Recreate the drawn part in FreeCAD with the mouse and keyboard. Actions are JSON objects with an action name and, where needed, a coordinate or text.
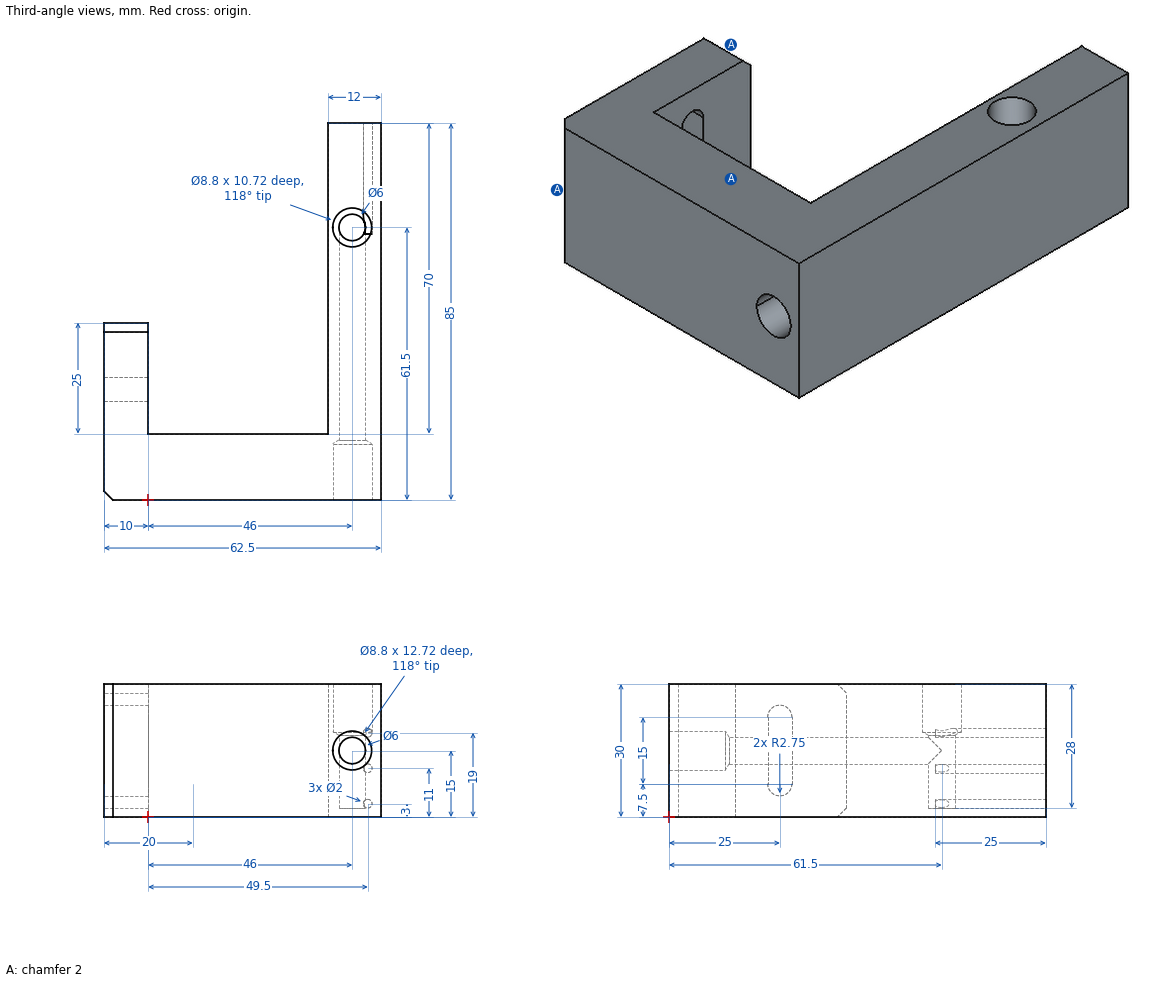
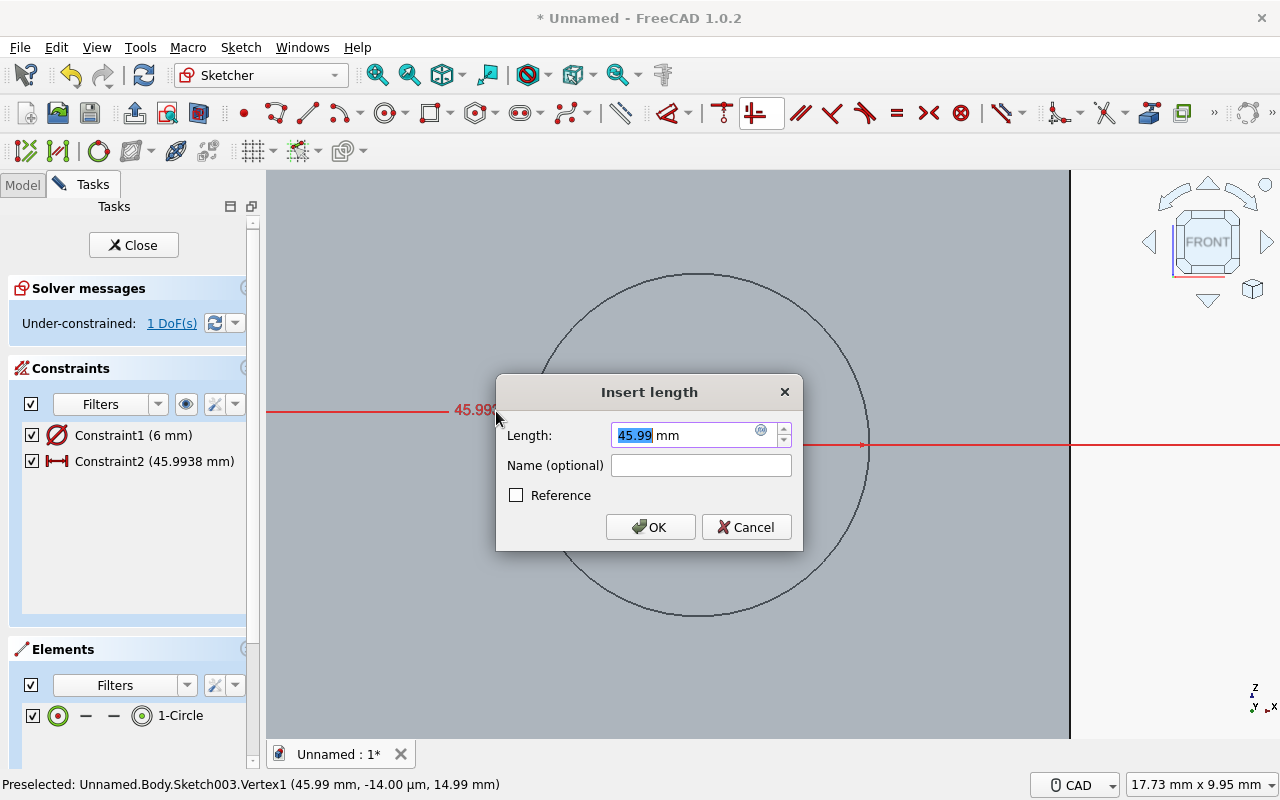
{"action": "type", "text": "46"}
{"action": "key", "text": "Return"}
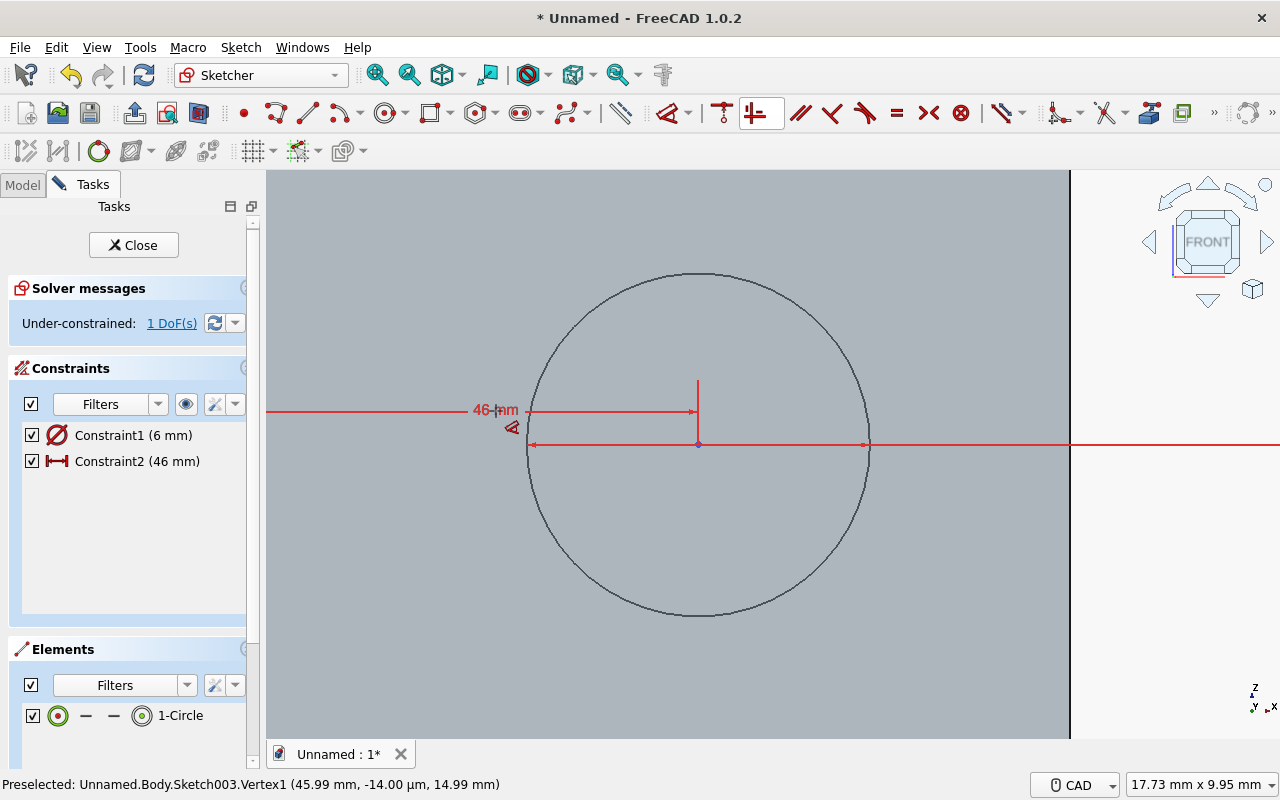
{"action": "left_click", "coordinate": [698, 445]}
{"action": "left_click", "coordinate": [732, 578]}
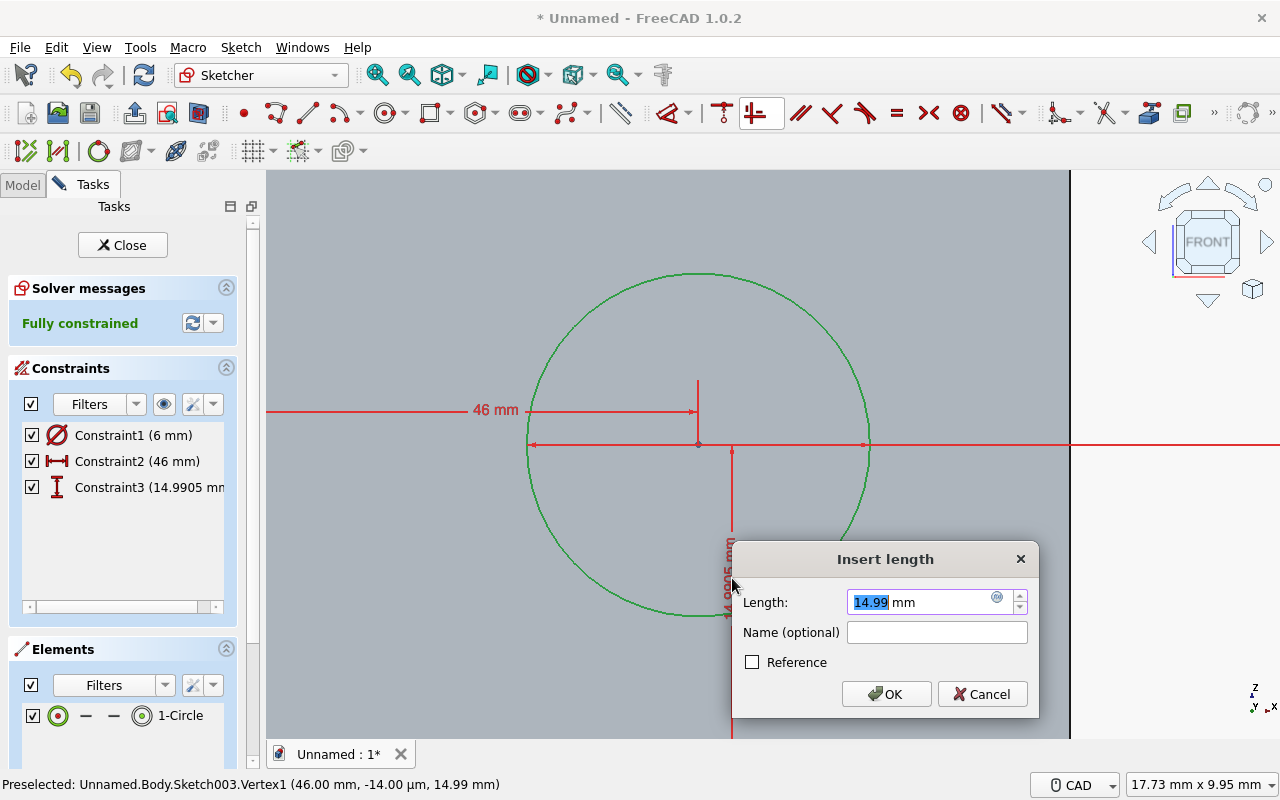
{"action": "type", "text": "15"}
{"action": "key", "text": "Return"}
{"action": "key", "text": "Escape"}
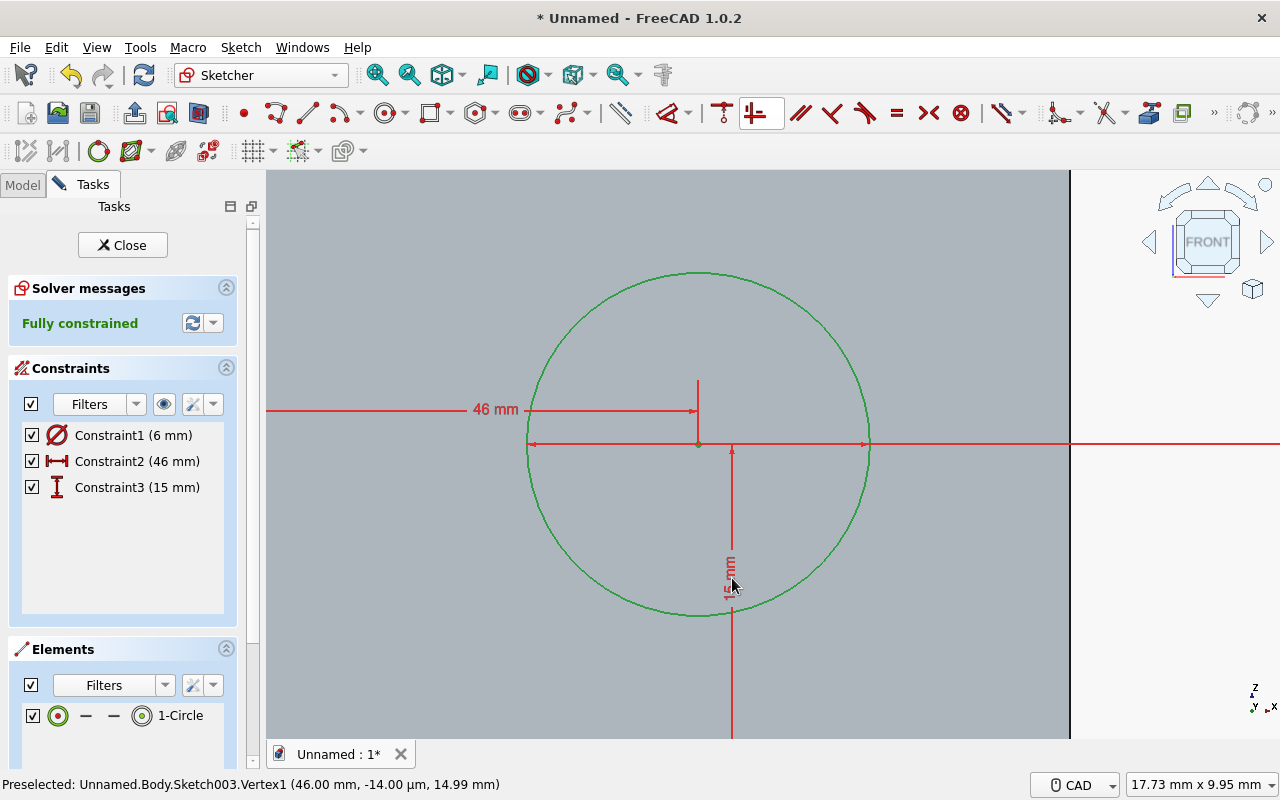
{"action": "left_click", "coordinate": [123, 245]}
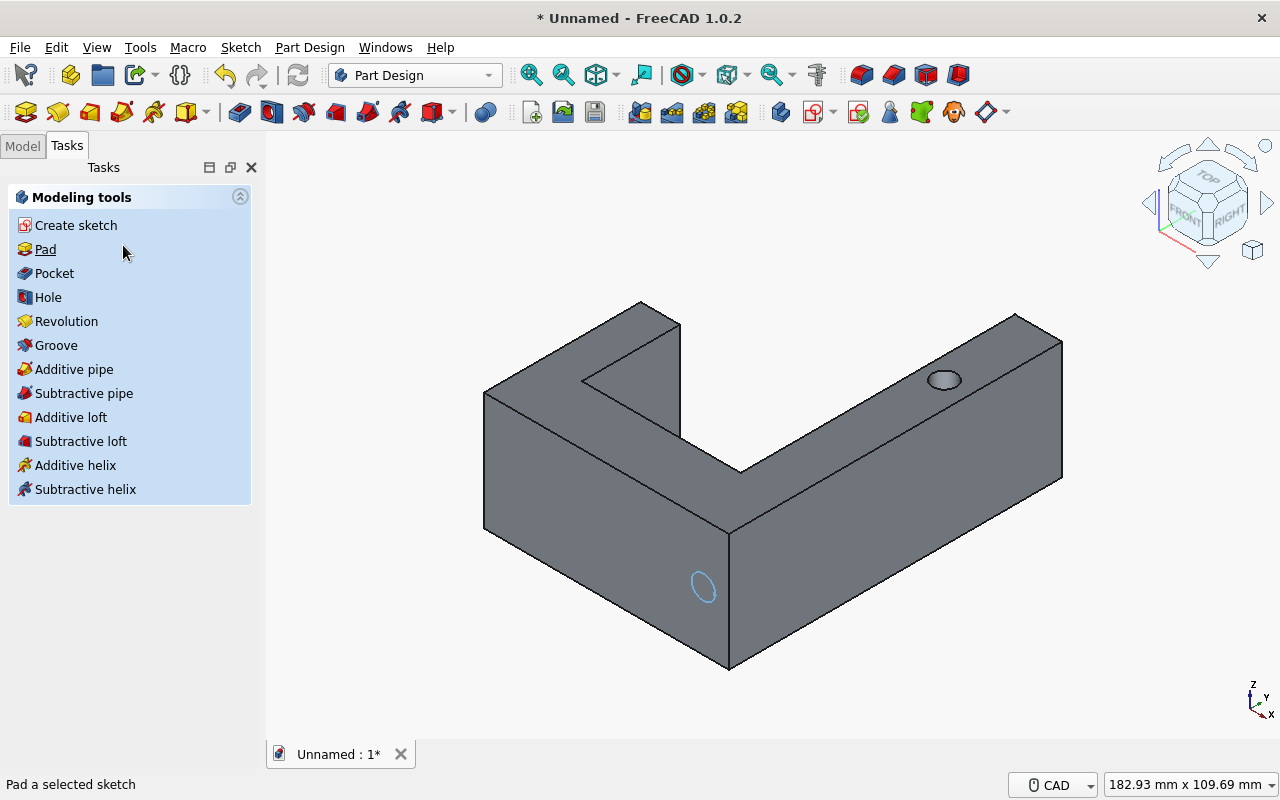
{"action": "left_click", "coordinate": [240, 112]}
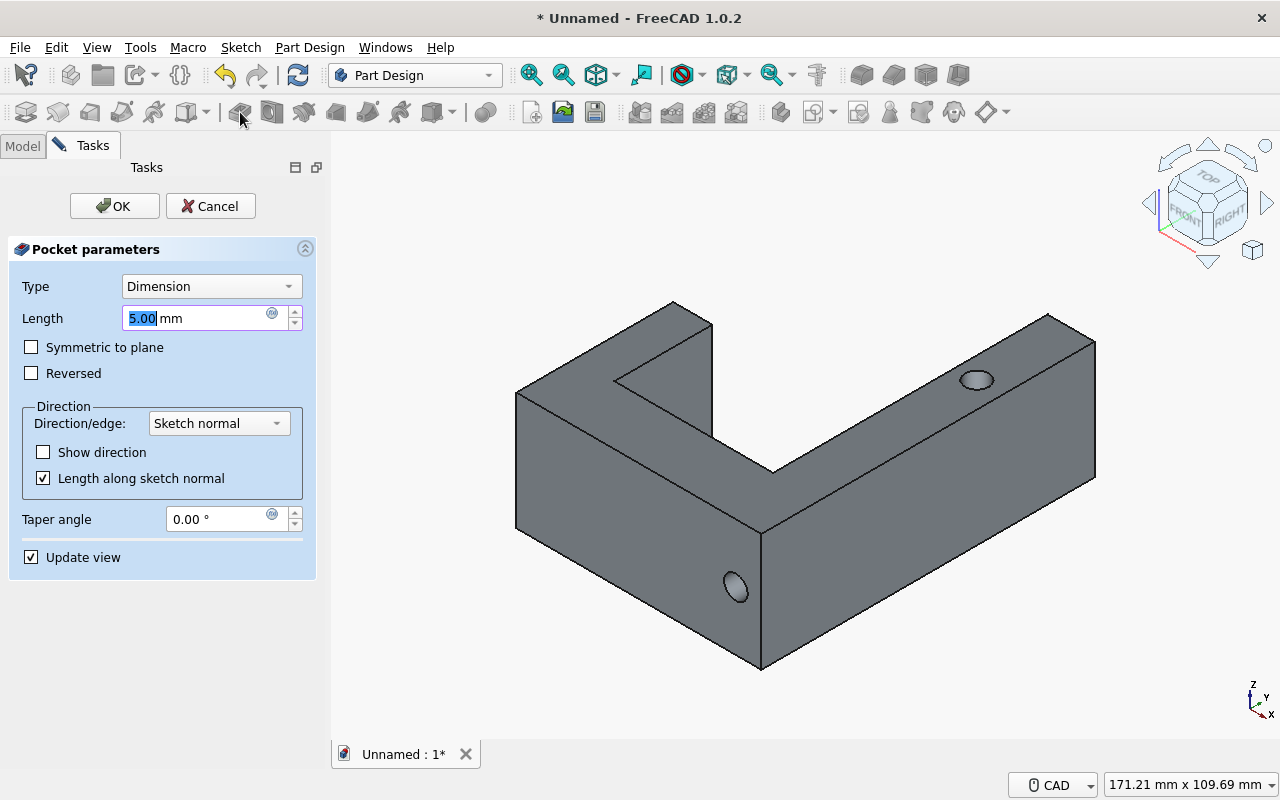
{"action": "type", "text": "61.5"}
{"action": "key", "text": "Tab"}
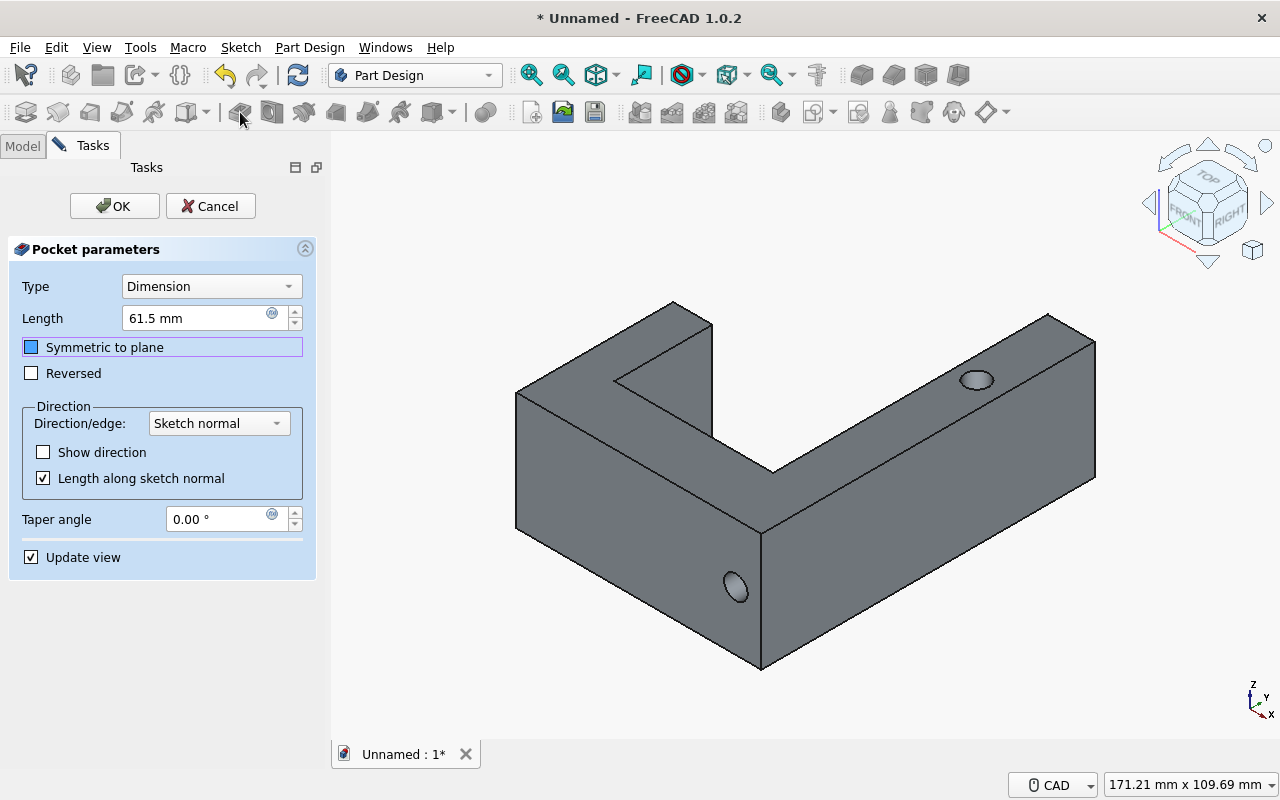
{"action": "left_click", "coordinate": [115, 206]}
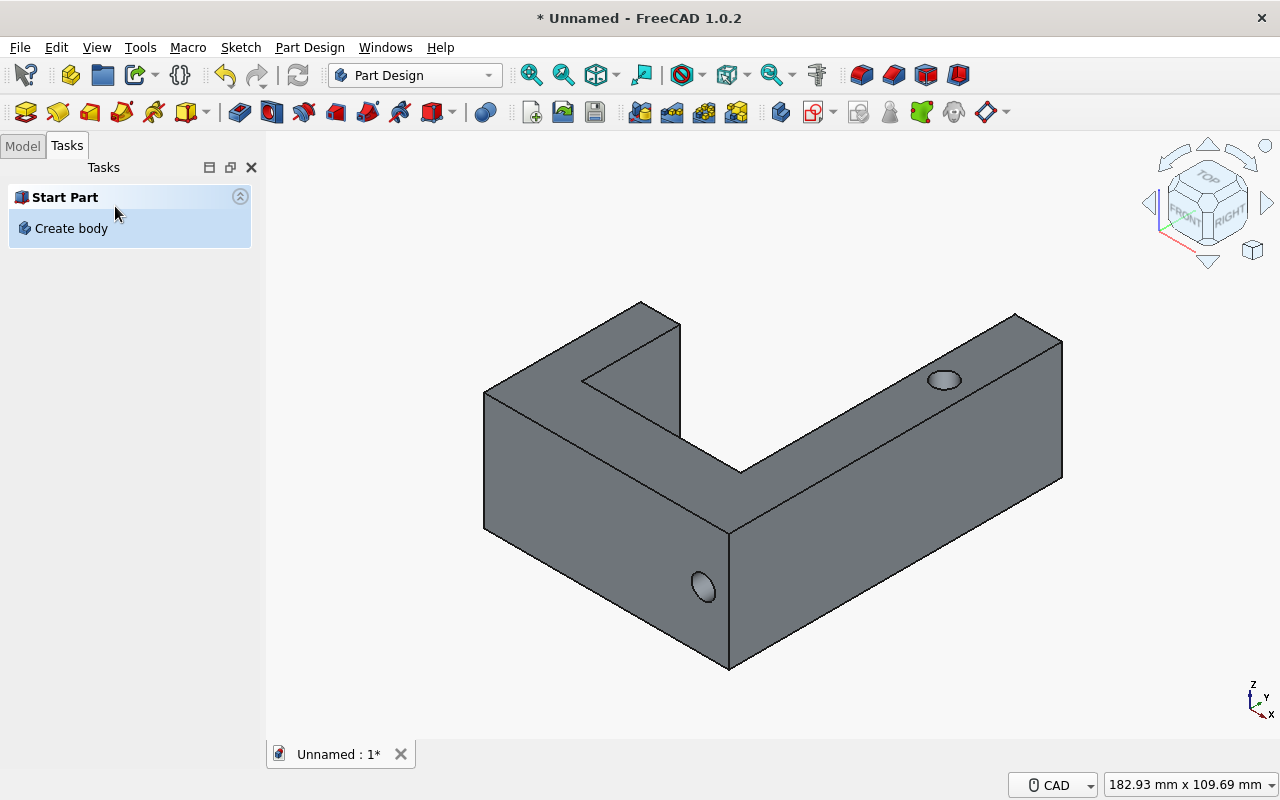
{"action": "key", "text": "6"}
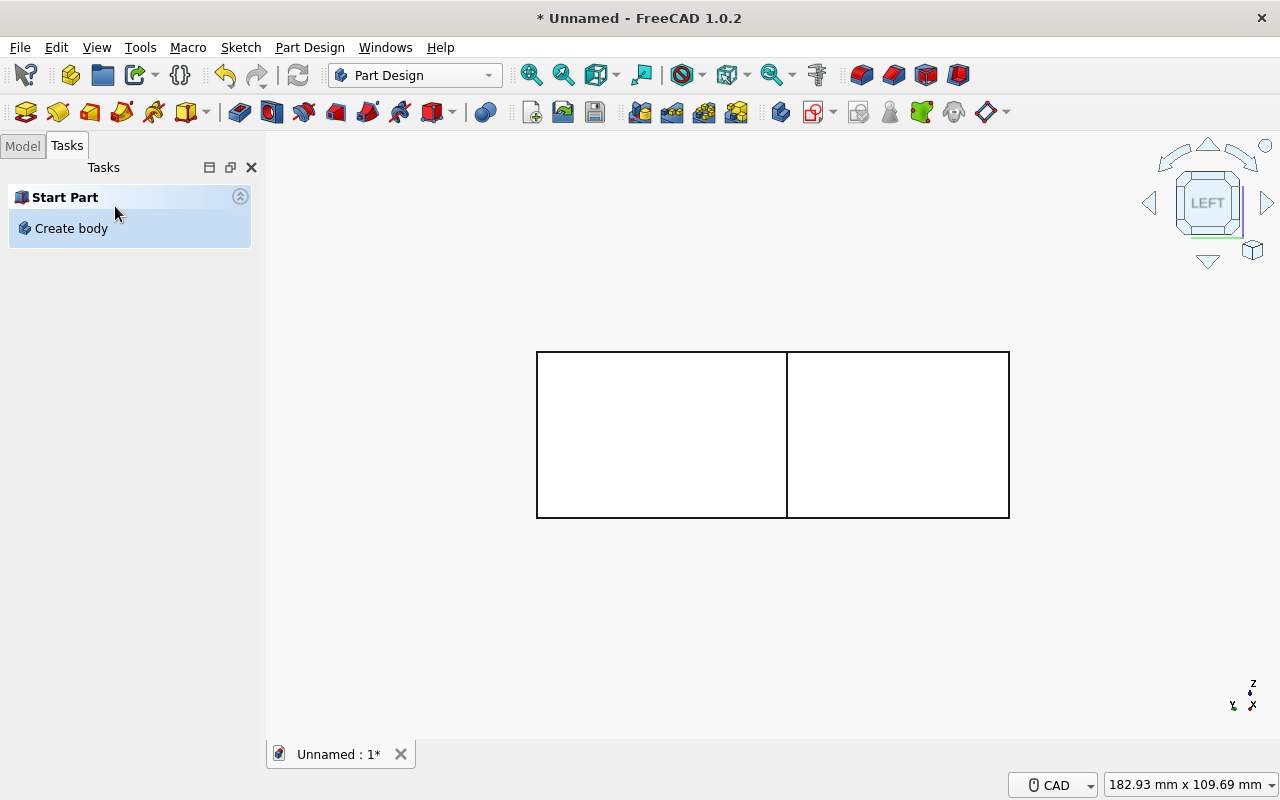
{"action": "left_click", "coordinate": [898, 434]}